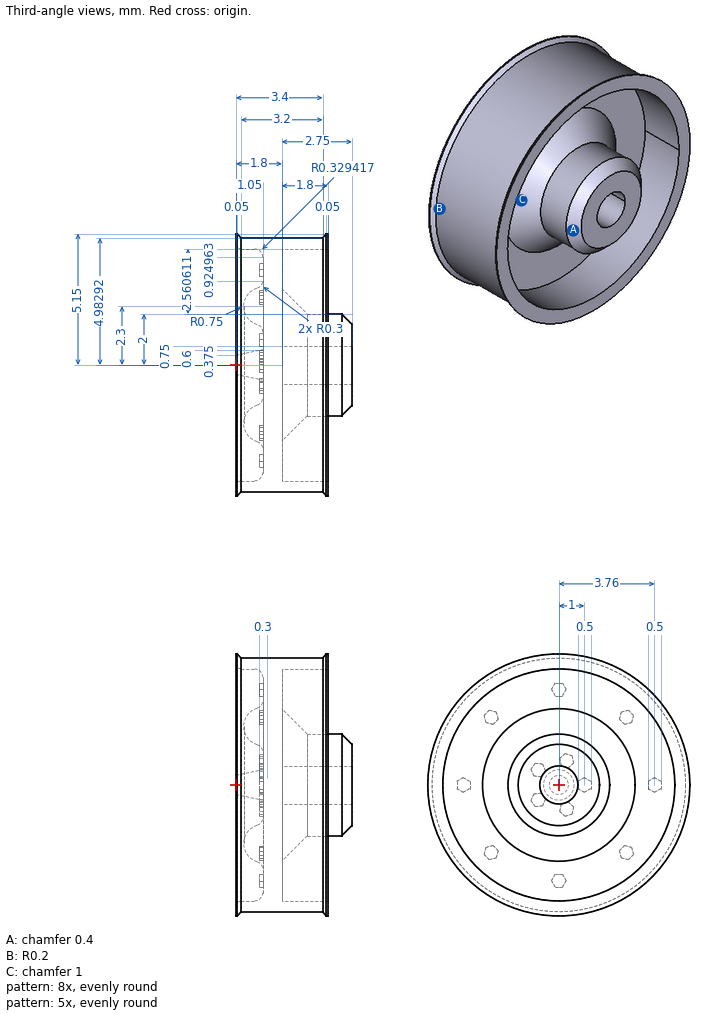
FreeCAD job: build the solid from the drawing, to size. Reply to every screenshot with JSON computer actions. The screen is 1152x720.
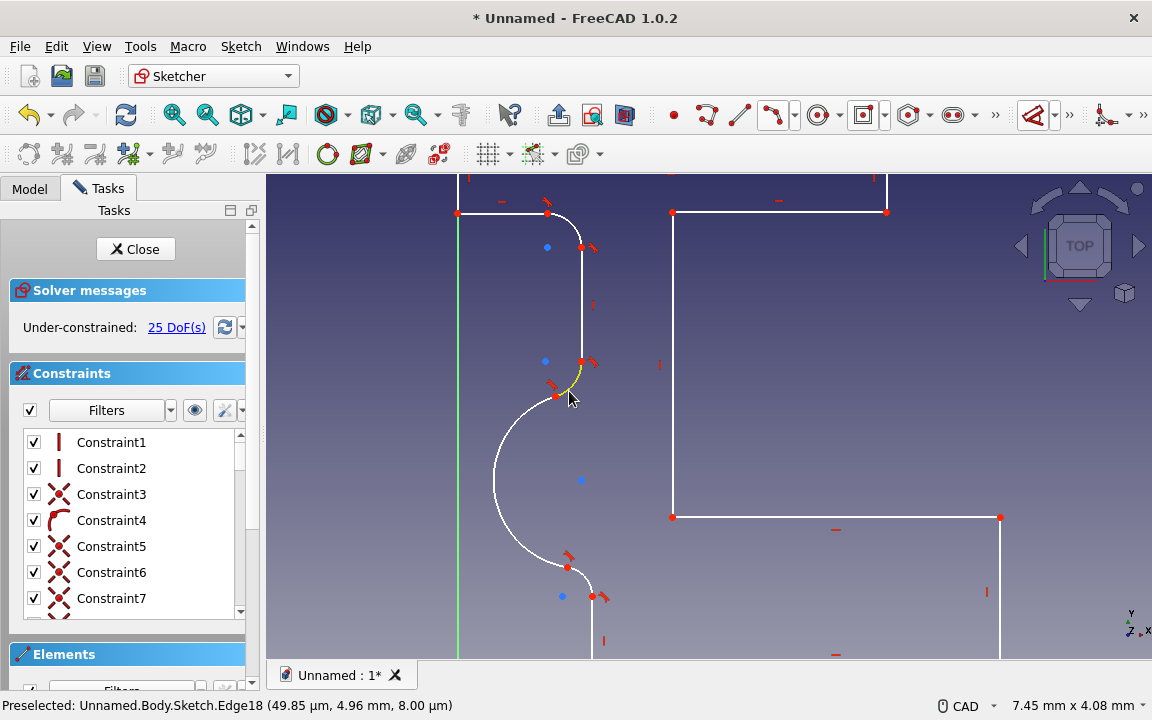
{"action": "left_click", "coordinate": [568, 390]}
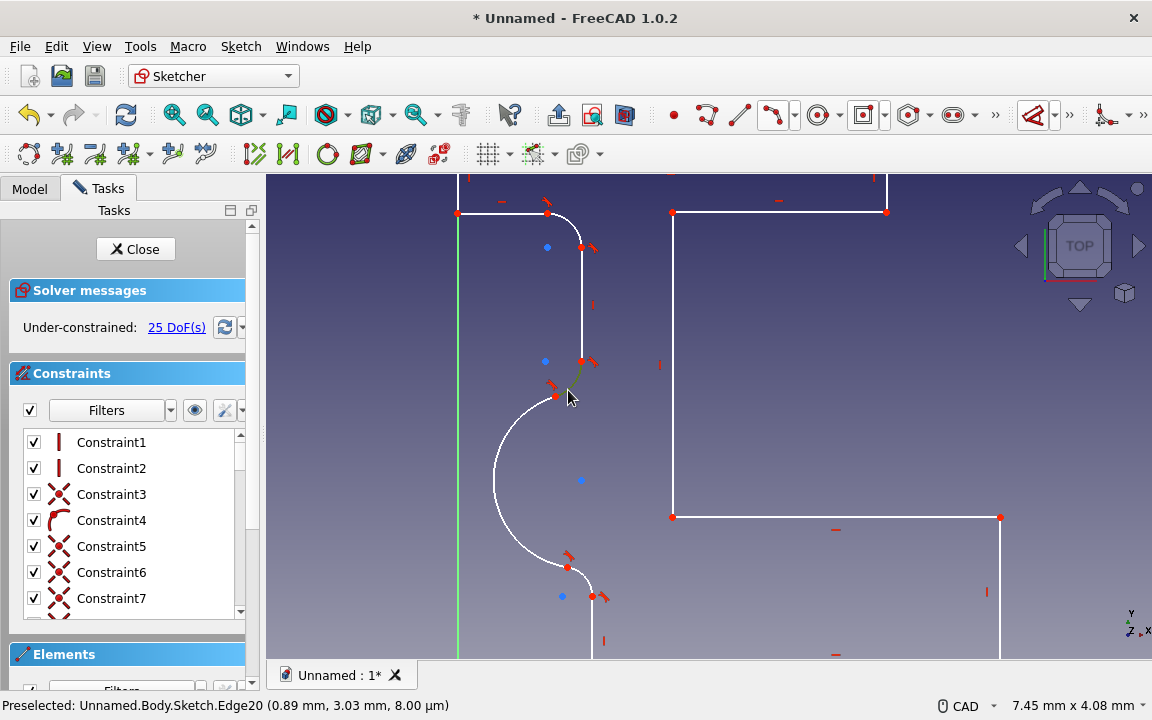
{"action": "left_click", "coordinate": [590, 584]}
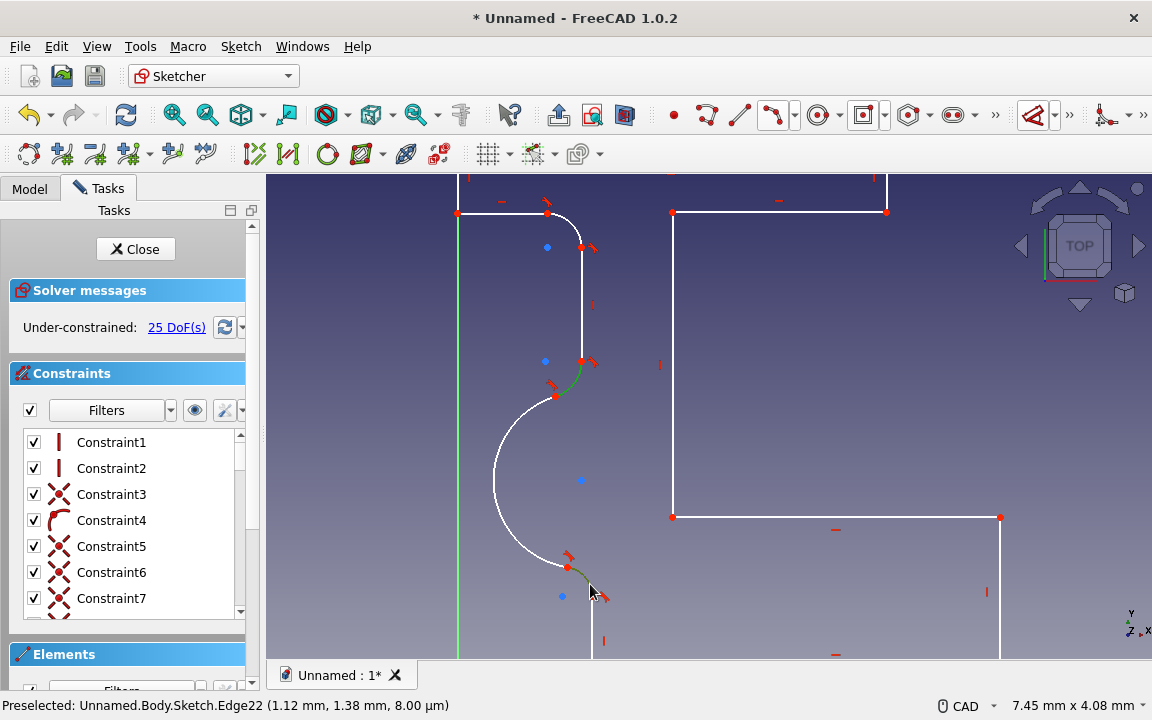
{"action": "key", "text": "e"}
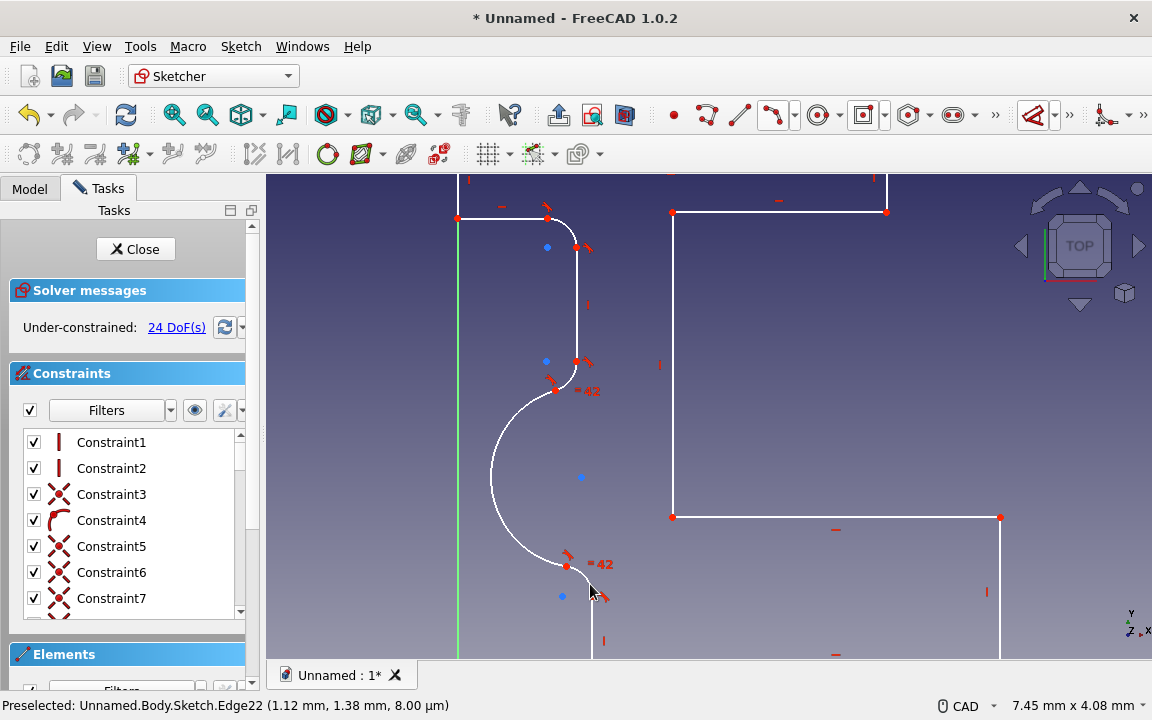
{"action": "left_click", "coordinate": [1032, 116]}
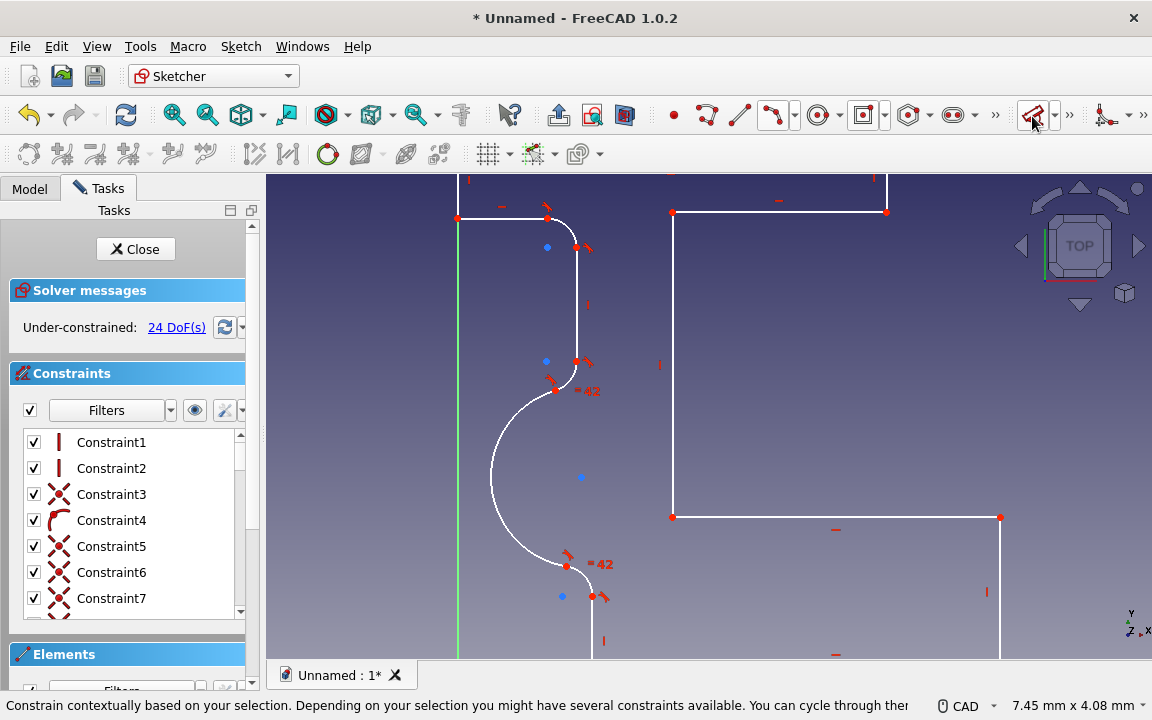
{"action": "left_click", "coordinate": [565, 385]}
{"action": "left_click", "coordinate": [585, 410]}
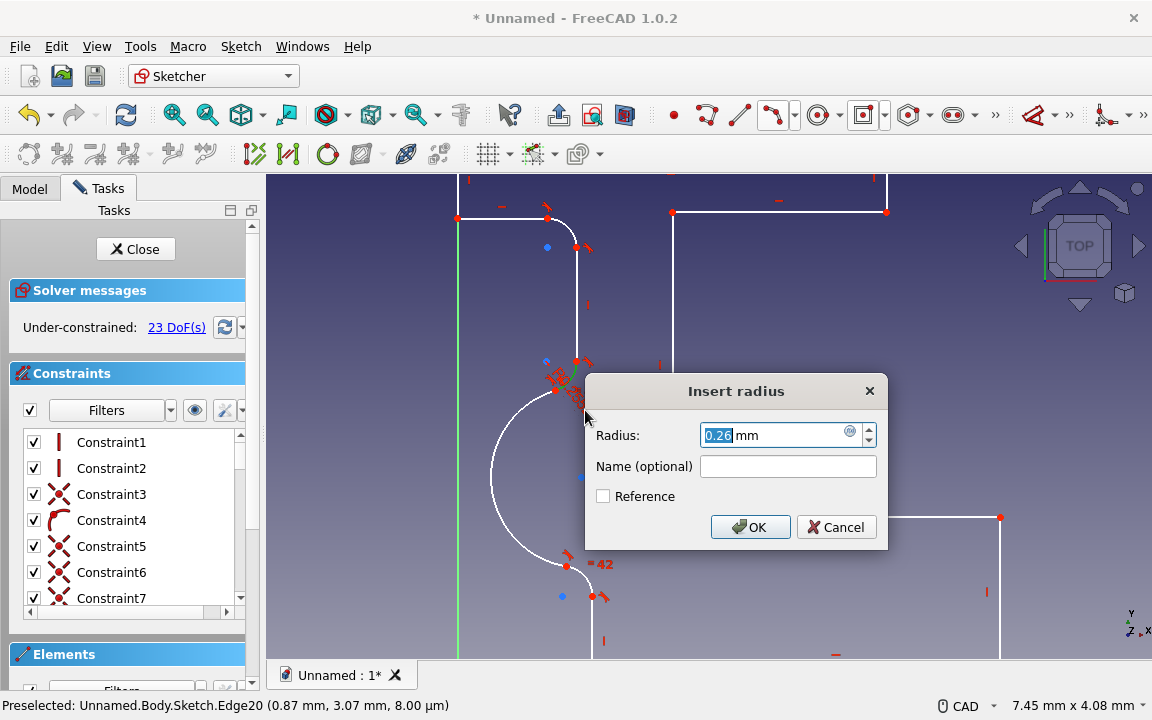
{"action": "type", "text": "0.3"}
{"action": "key", "text": "Return"}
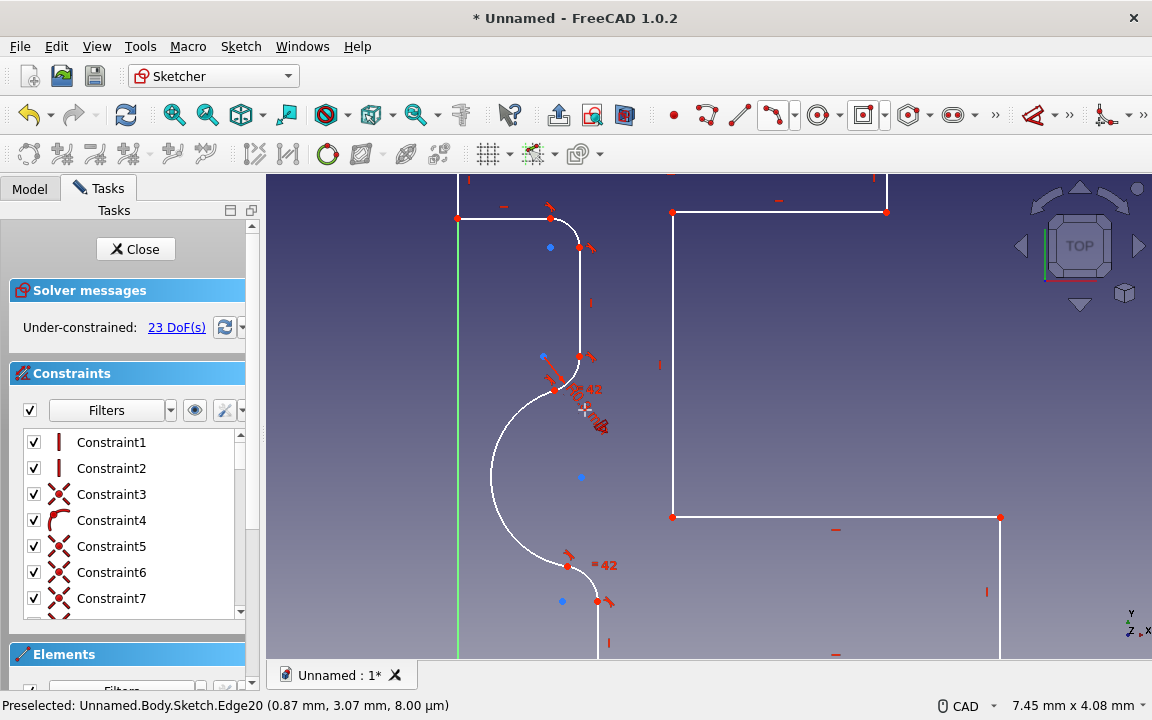
{"action": "left_click", "coordinate": [501, 437]}
{"action": "left_click", "coordinate": [472, 423]}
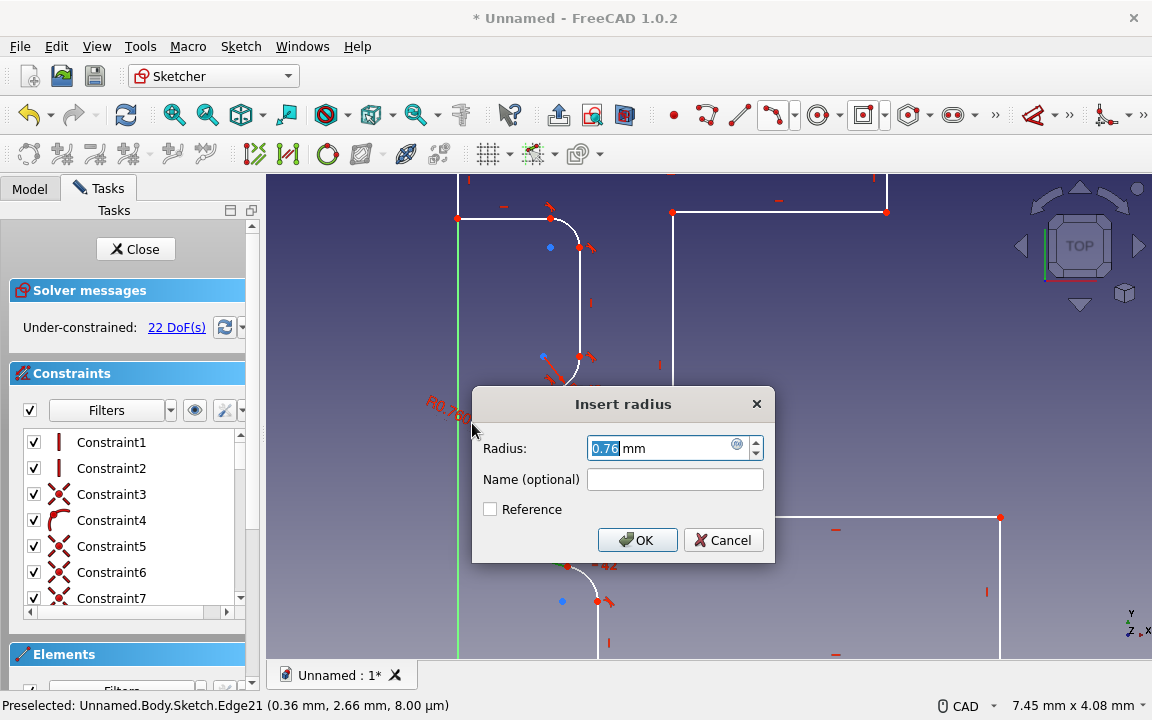
{"action": "type", "text": "0.75"}
{"action": "key", "text": "Return"}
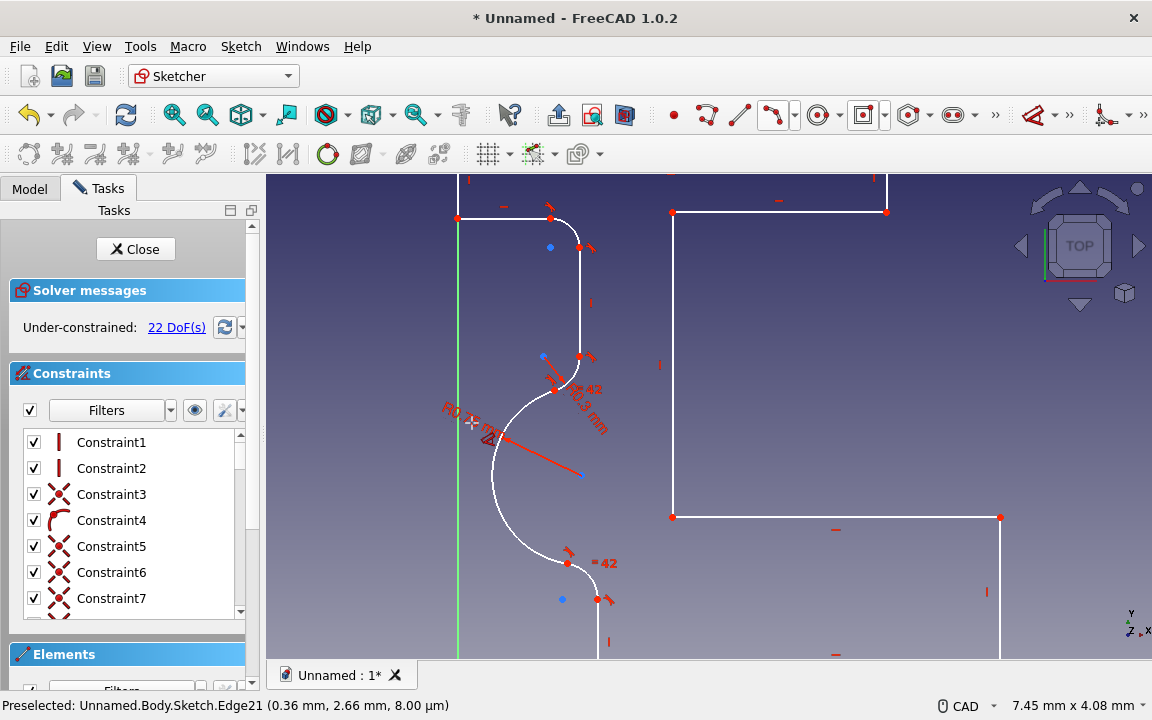
{"action": "left_click", "coordinate": [576, 235]}
{"action": "left_click", "coordinate": [605, 221]}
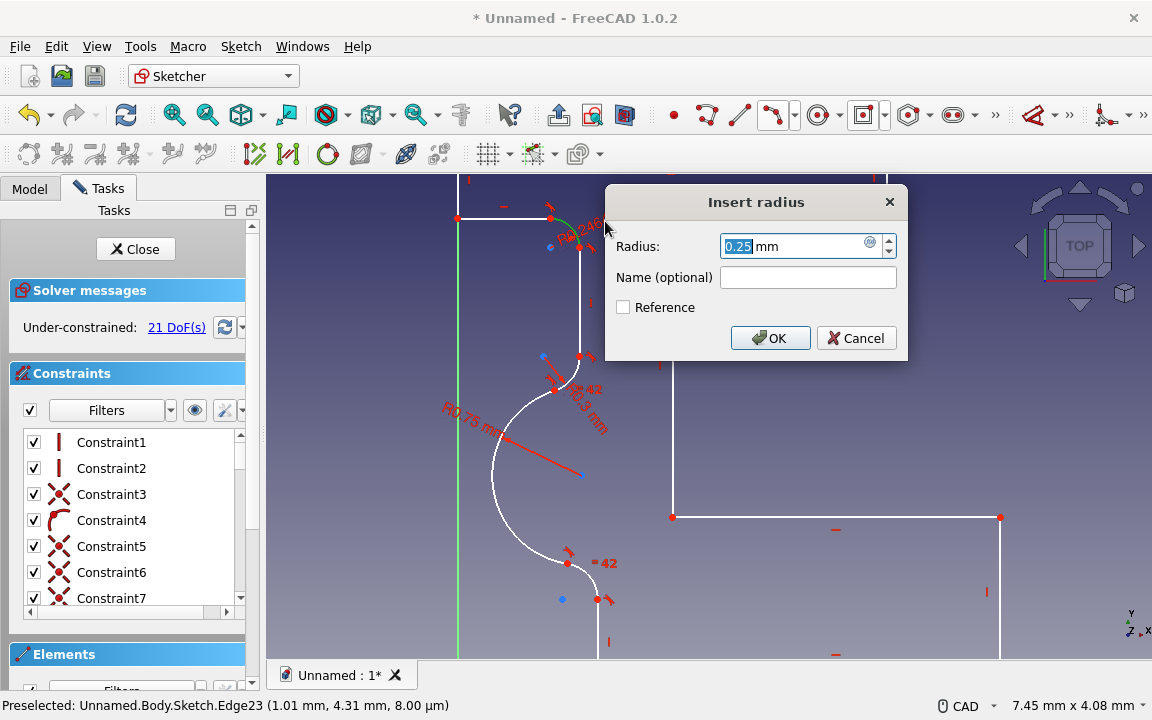
{"action": "type", "text": "0.329417"}
{"action": "key", "text": "Return"}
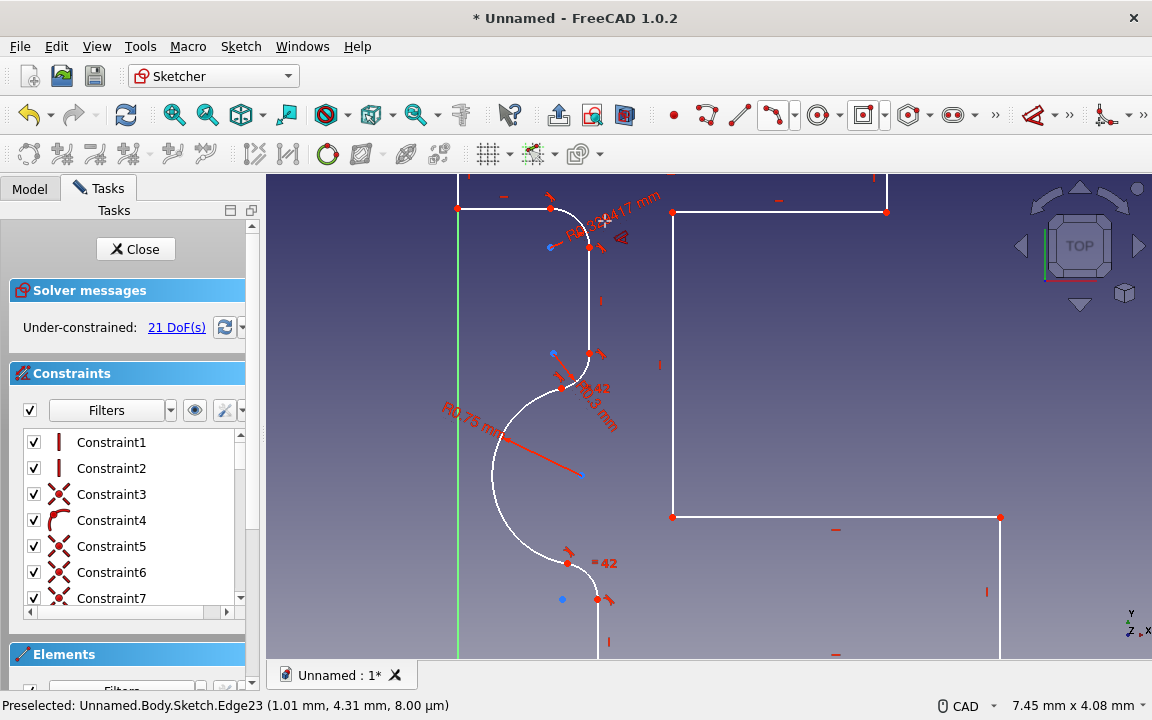
{"action": "scroll", "coordinate": [569, 392], "scroll_direction": "down", "scroll_amount": 4}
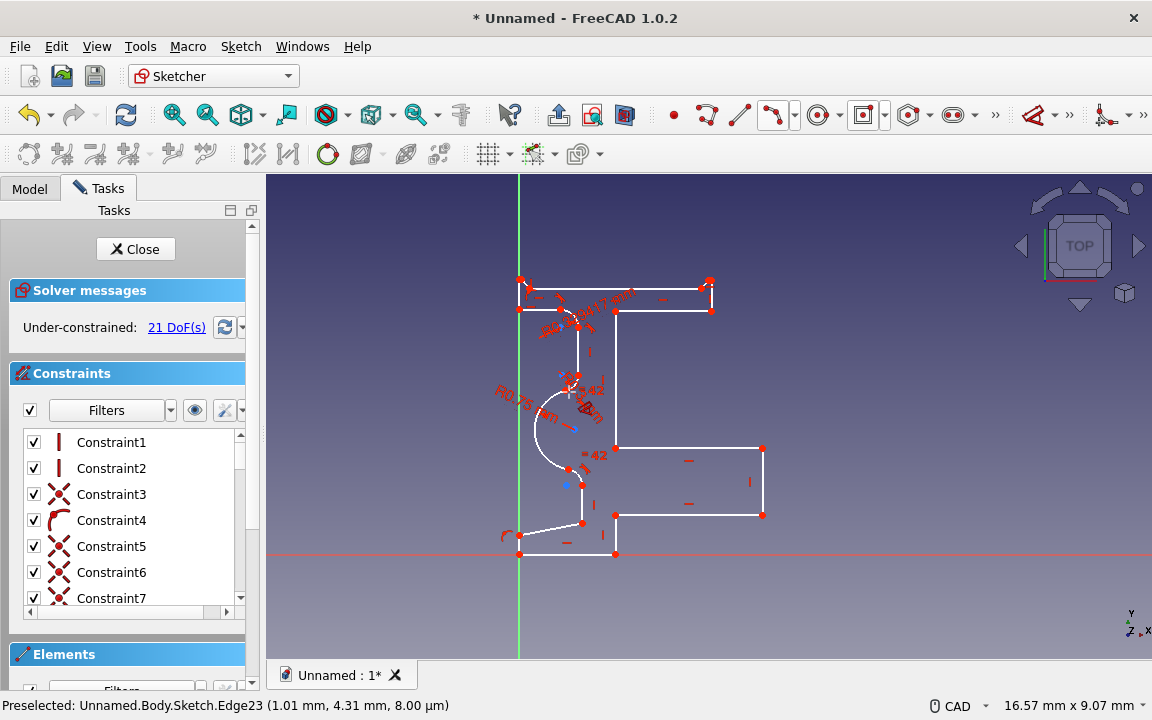
{"action": "left_click", "coordinate": [763, 448]}
{"action": "left_click", "coordinate": [797, 501]}